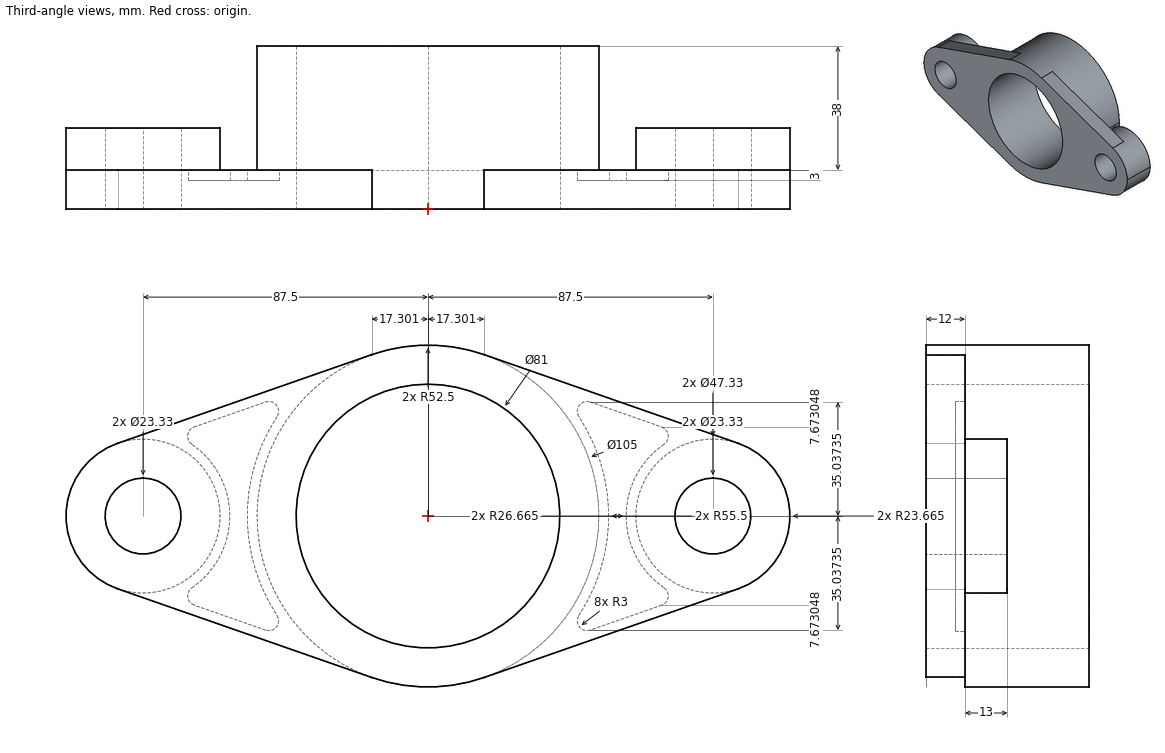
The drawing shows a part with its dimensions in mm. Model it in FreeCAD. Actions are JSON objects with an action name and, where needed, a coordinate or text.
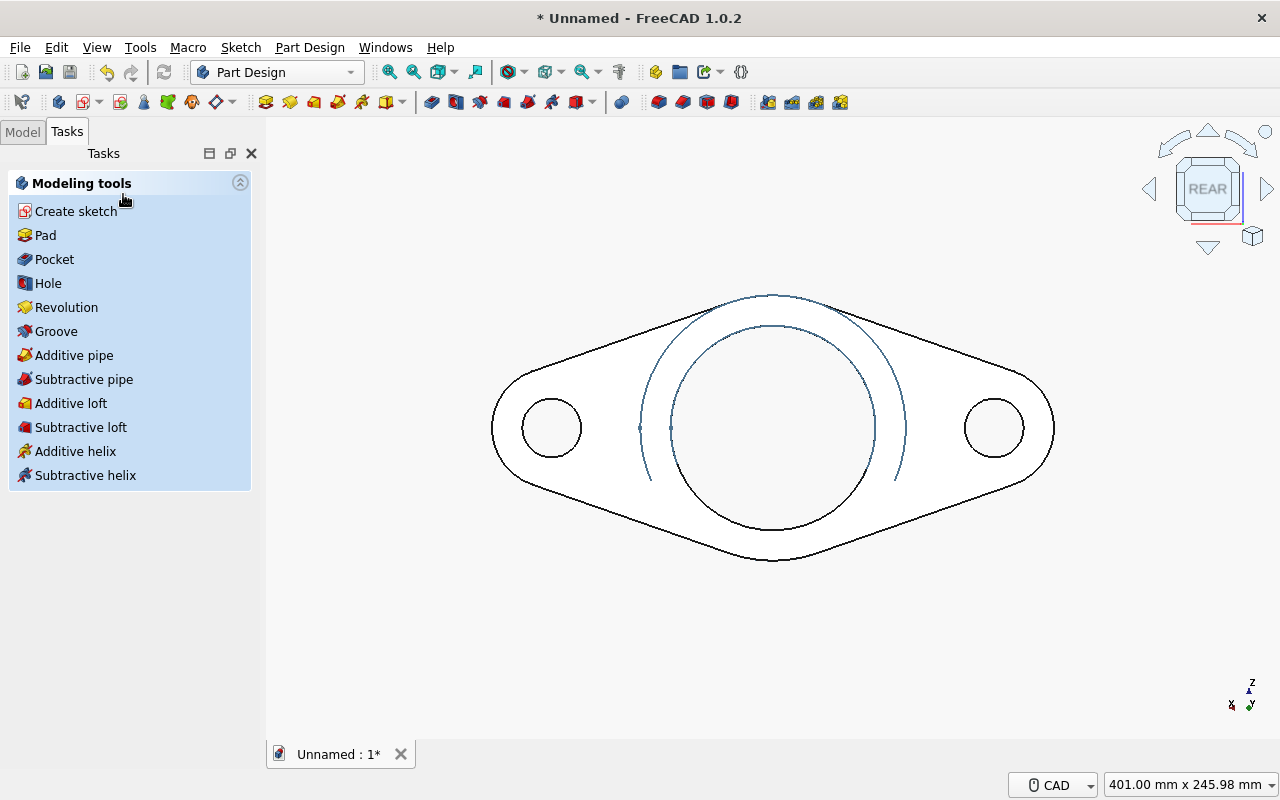
{"action": "left_click", "coordinate": [266, 102]}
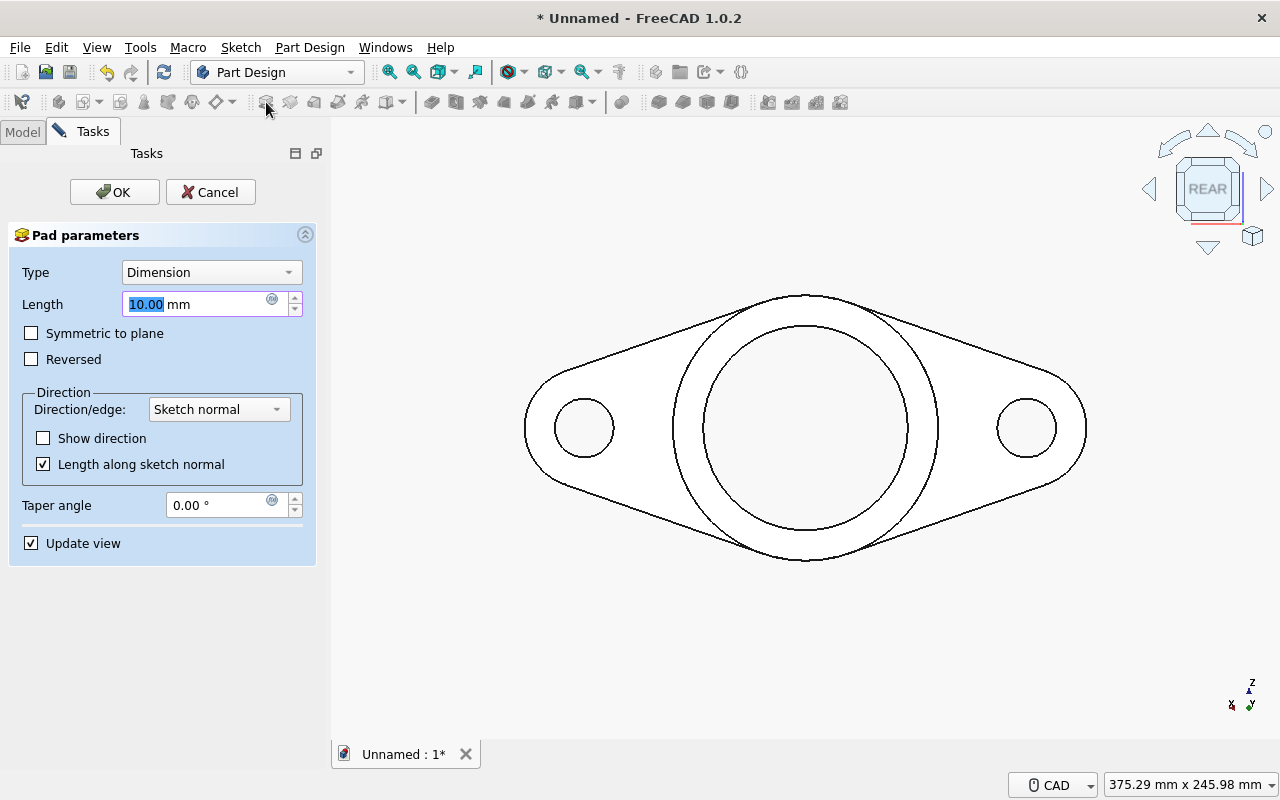
{"action": "type", "text": "38"}
{"action": "key", "text": "Tab"}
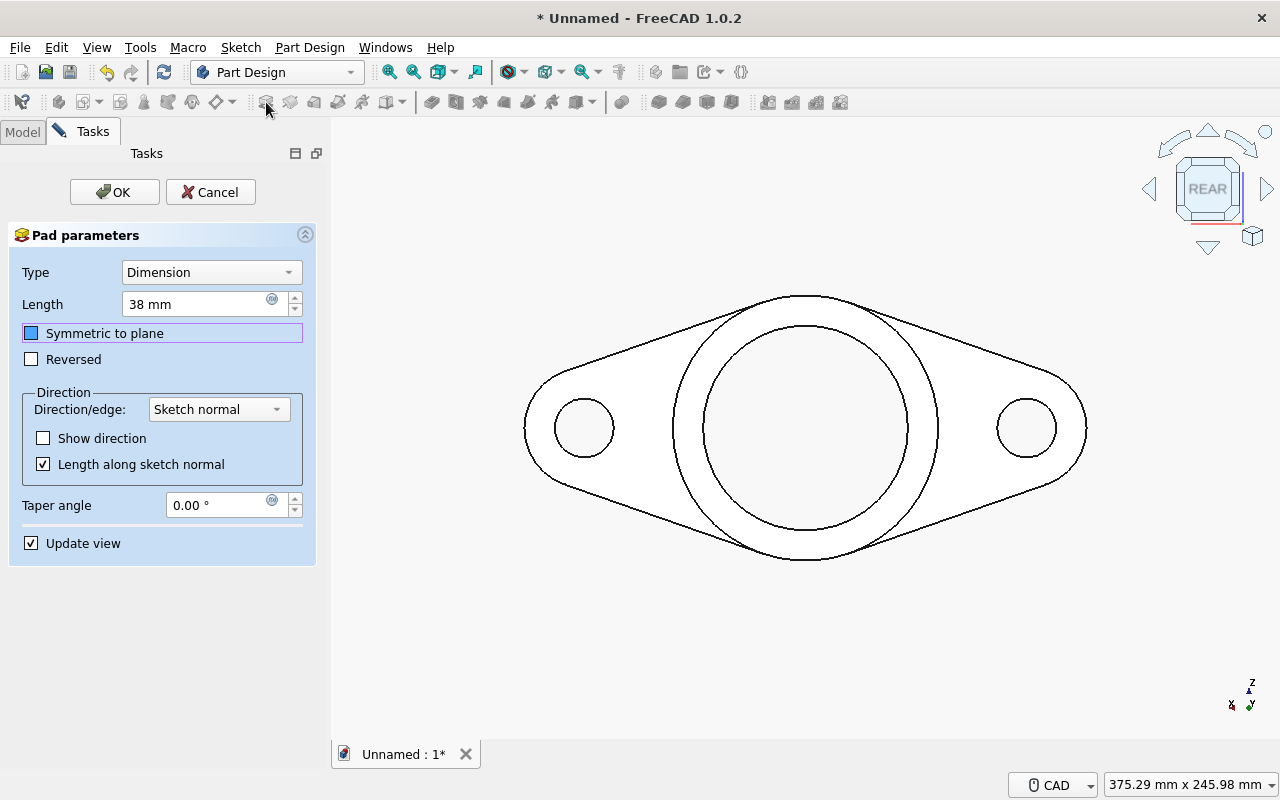
{"action": "left_click", "coordinate": [115, 192]}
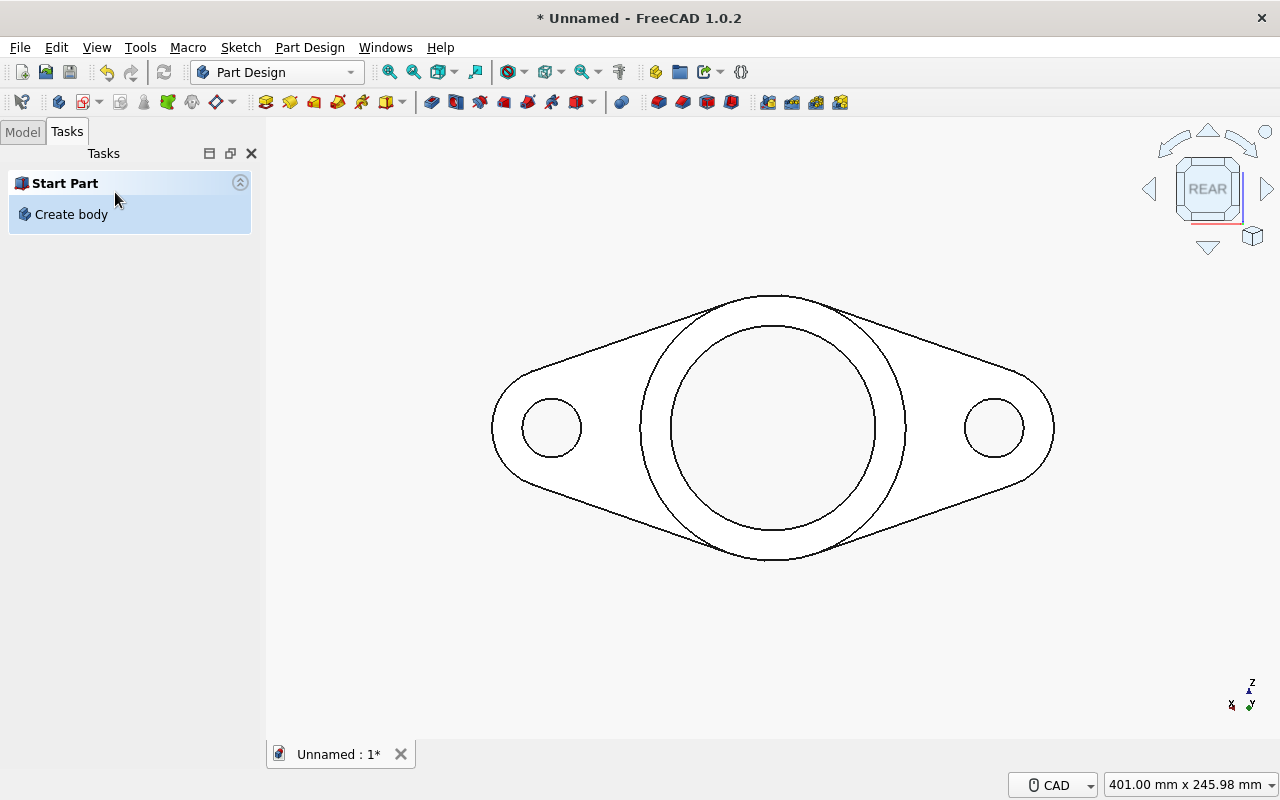
{"action": "left_click", "coordinate": [935, 463]}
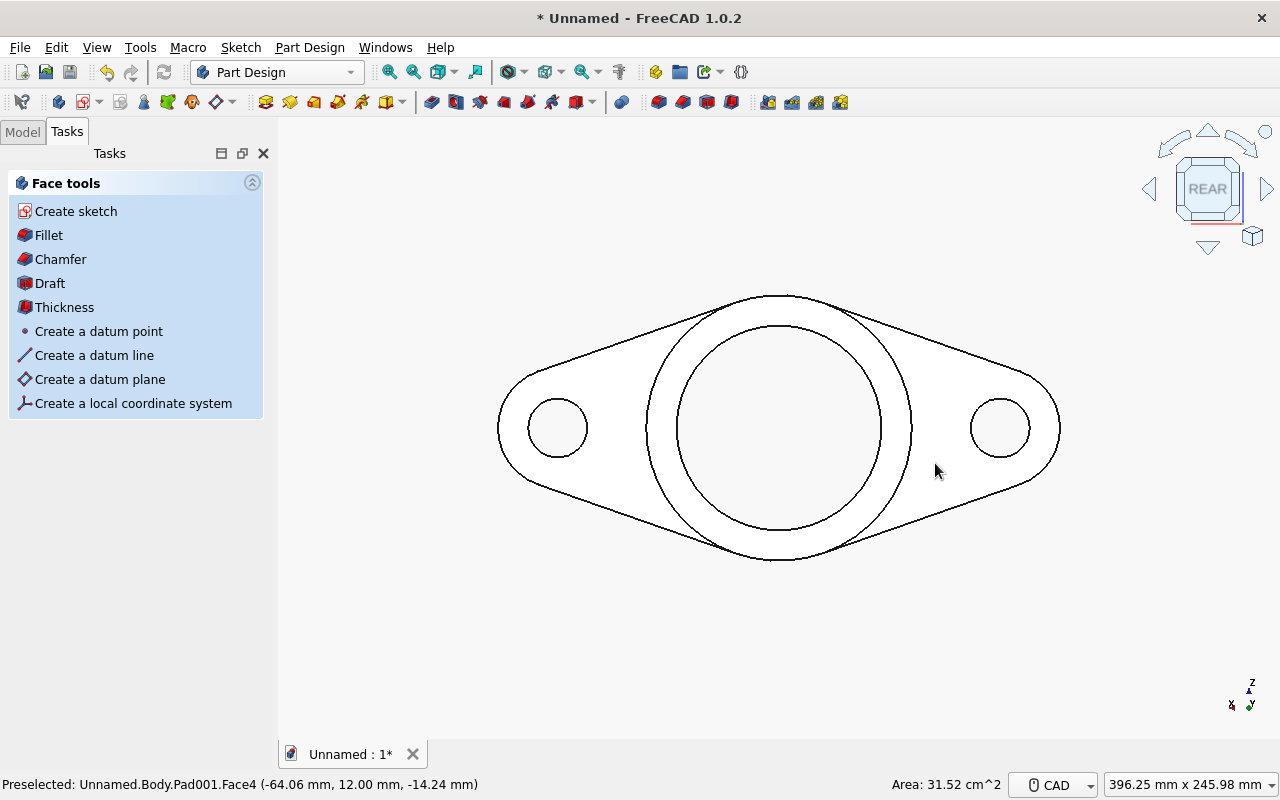
{"action": "left_click", "coordinate": [84, 102]}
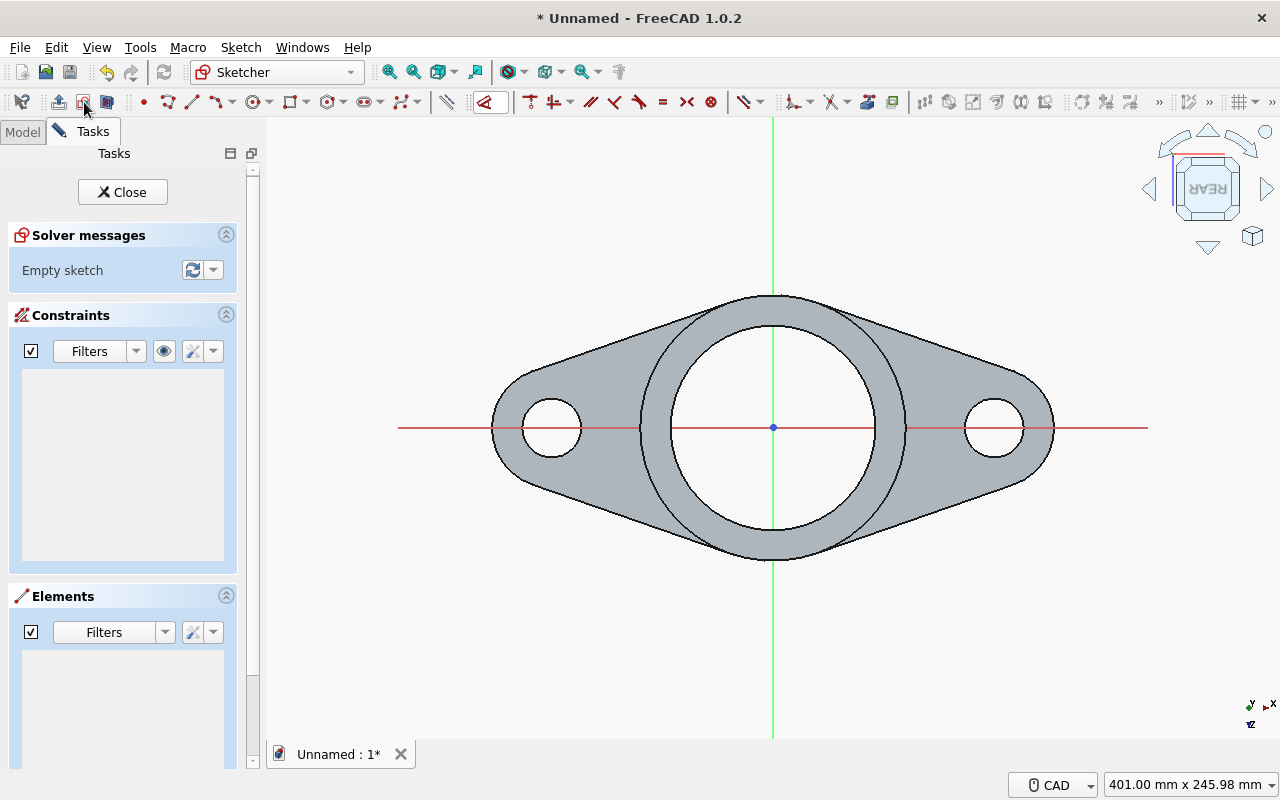
{"action": "left_click", "coordinate": [254, 102]}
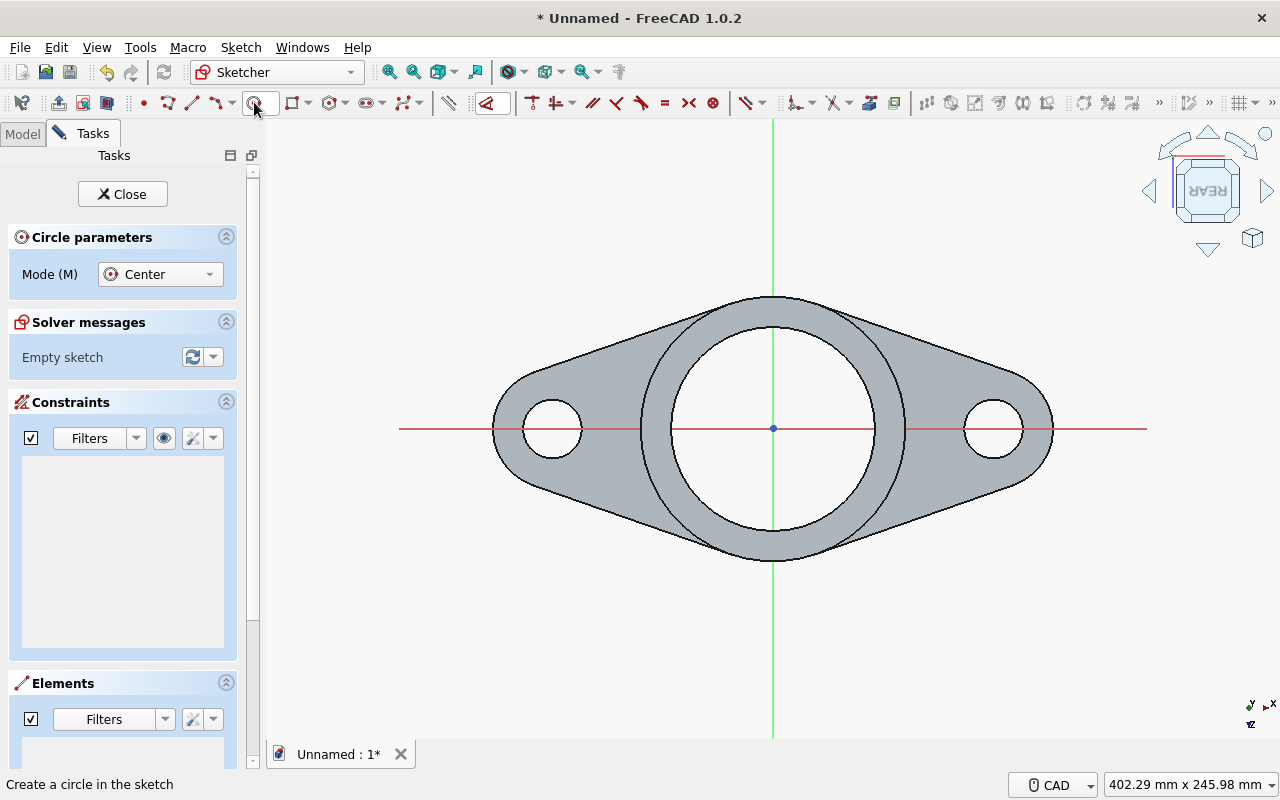
{"action": "left_click", "coordinate": [994, 429]}
{"action": "mouse_move", "coordinate": [1036, 387]}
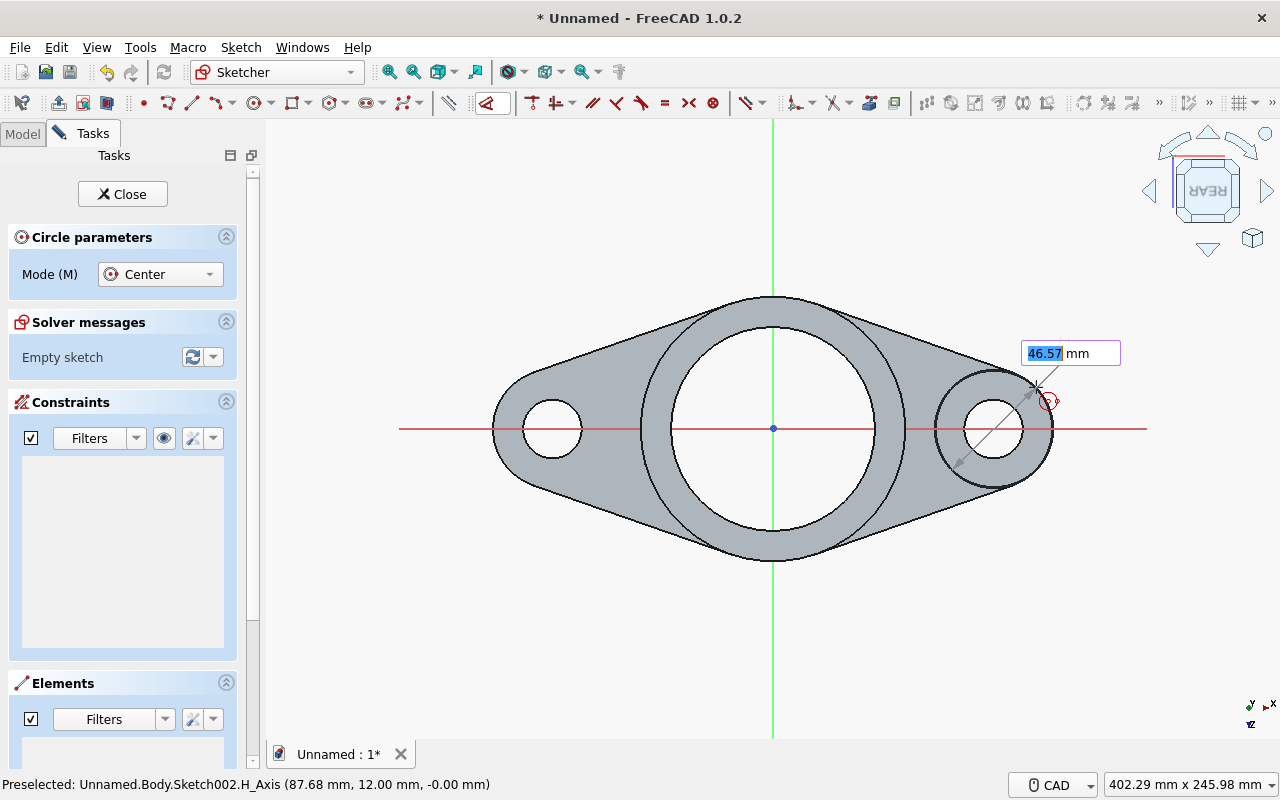
{"action": "type", "text": "47.33"}
{"action": "key", "text": "Return"}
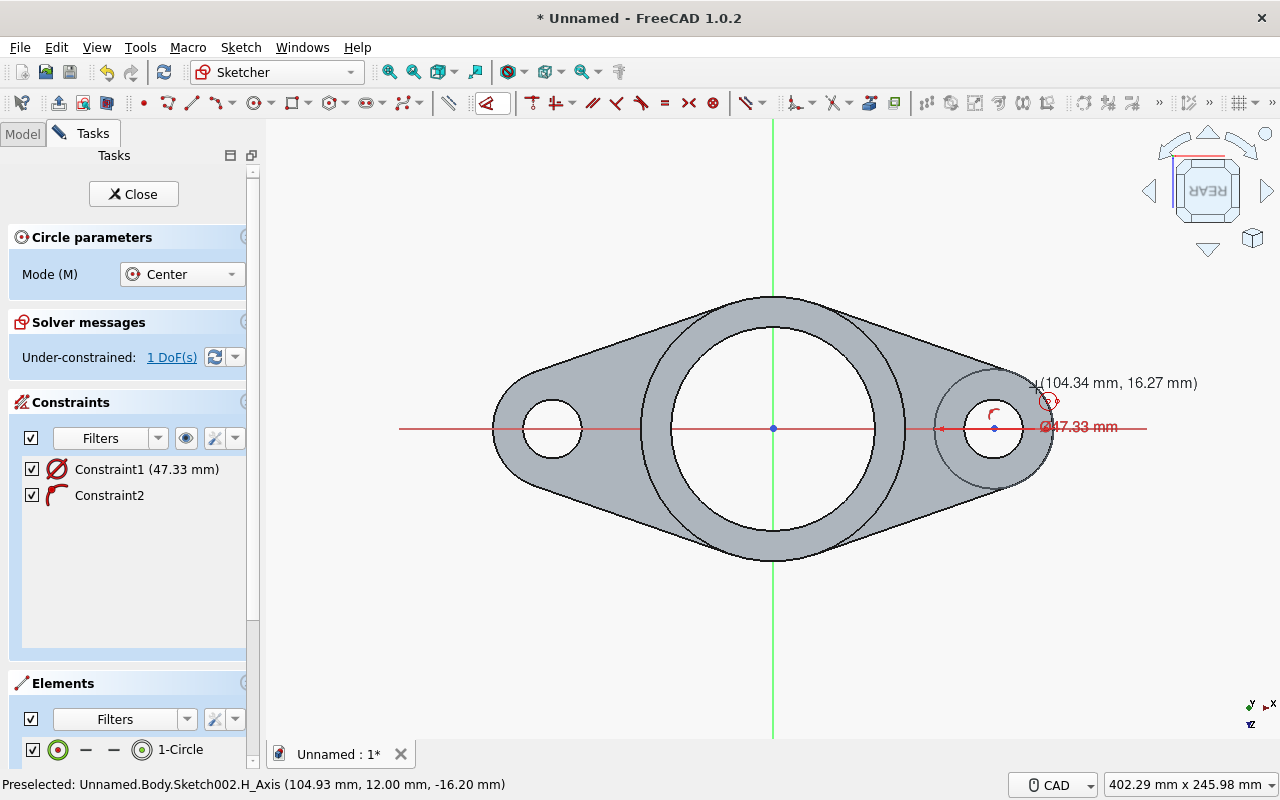
{"action": "left_click", "coordinate": [552, 429]}
{"action": "mouse_move", "coordinate": [595, 387]}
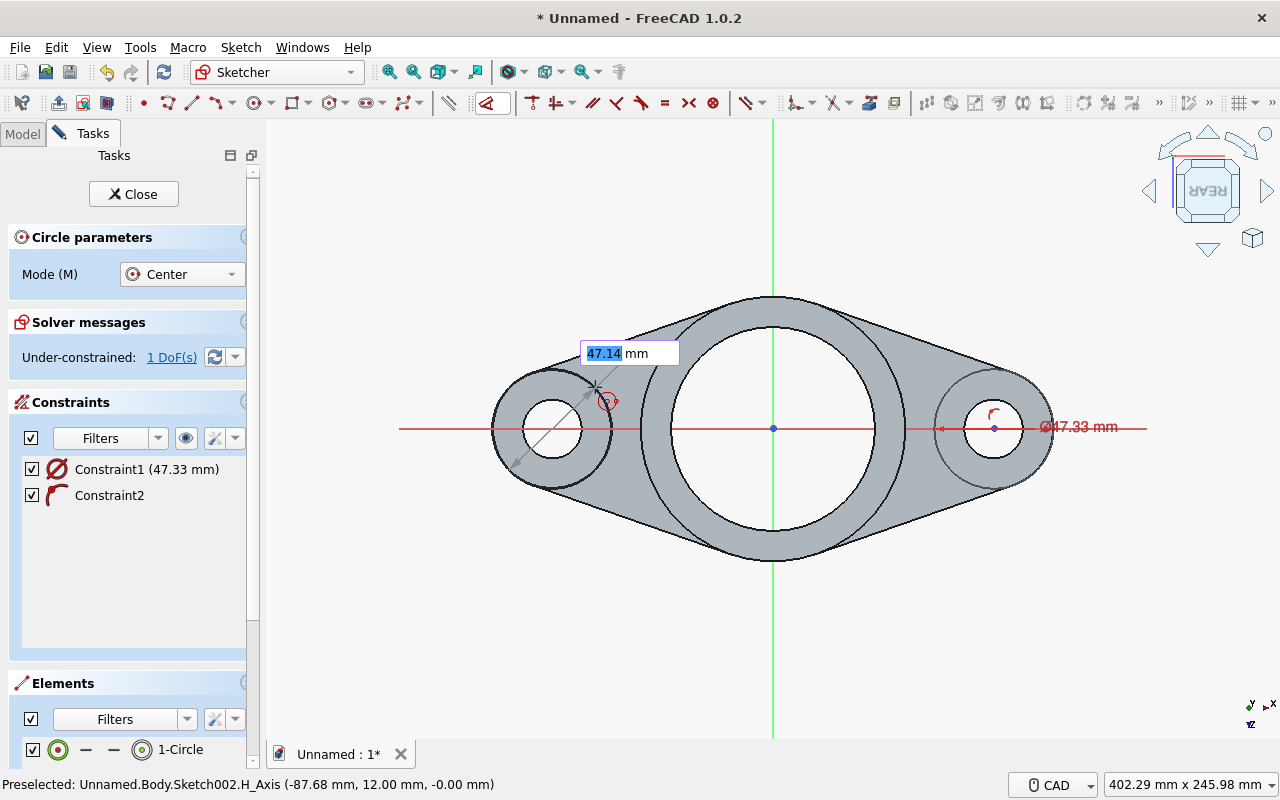
{"action": "type", "text": "47.33"}
{"action": "key", "text": "Return"}